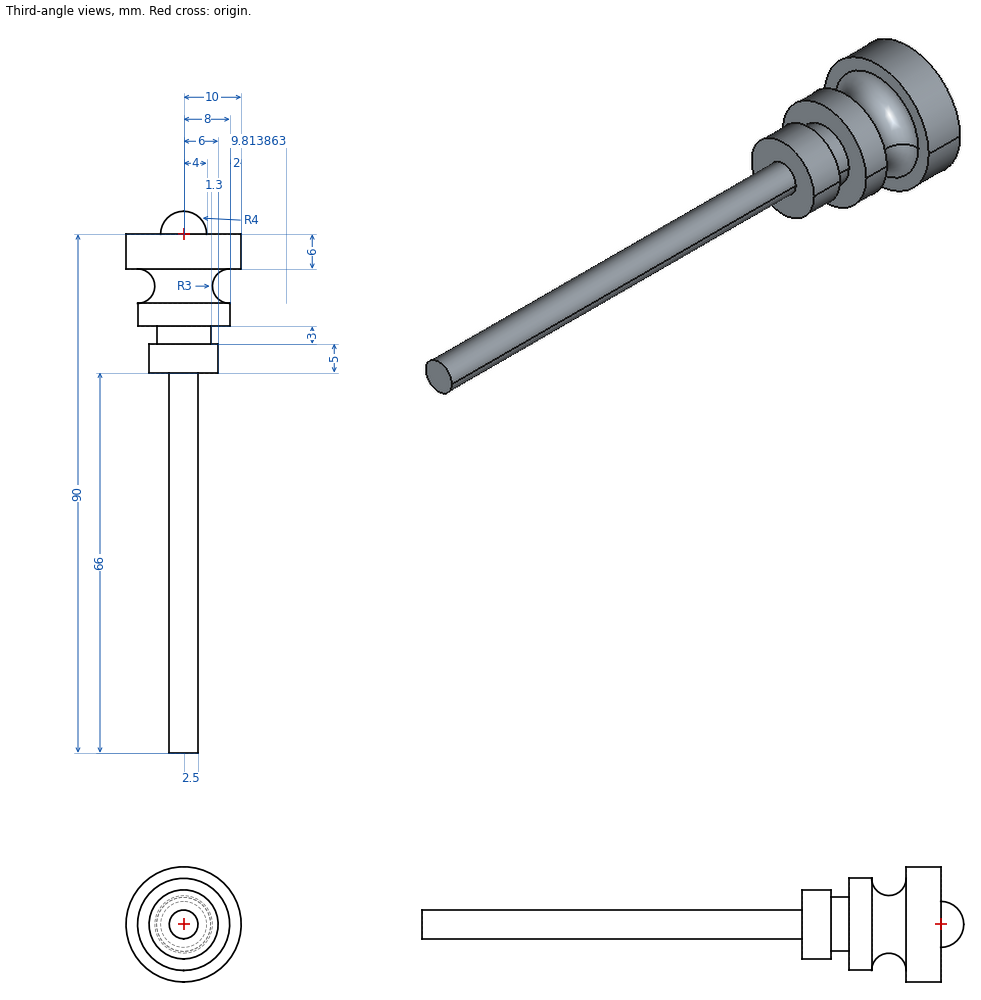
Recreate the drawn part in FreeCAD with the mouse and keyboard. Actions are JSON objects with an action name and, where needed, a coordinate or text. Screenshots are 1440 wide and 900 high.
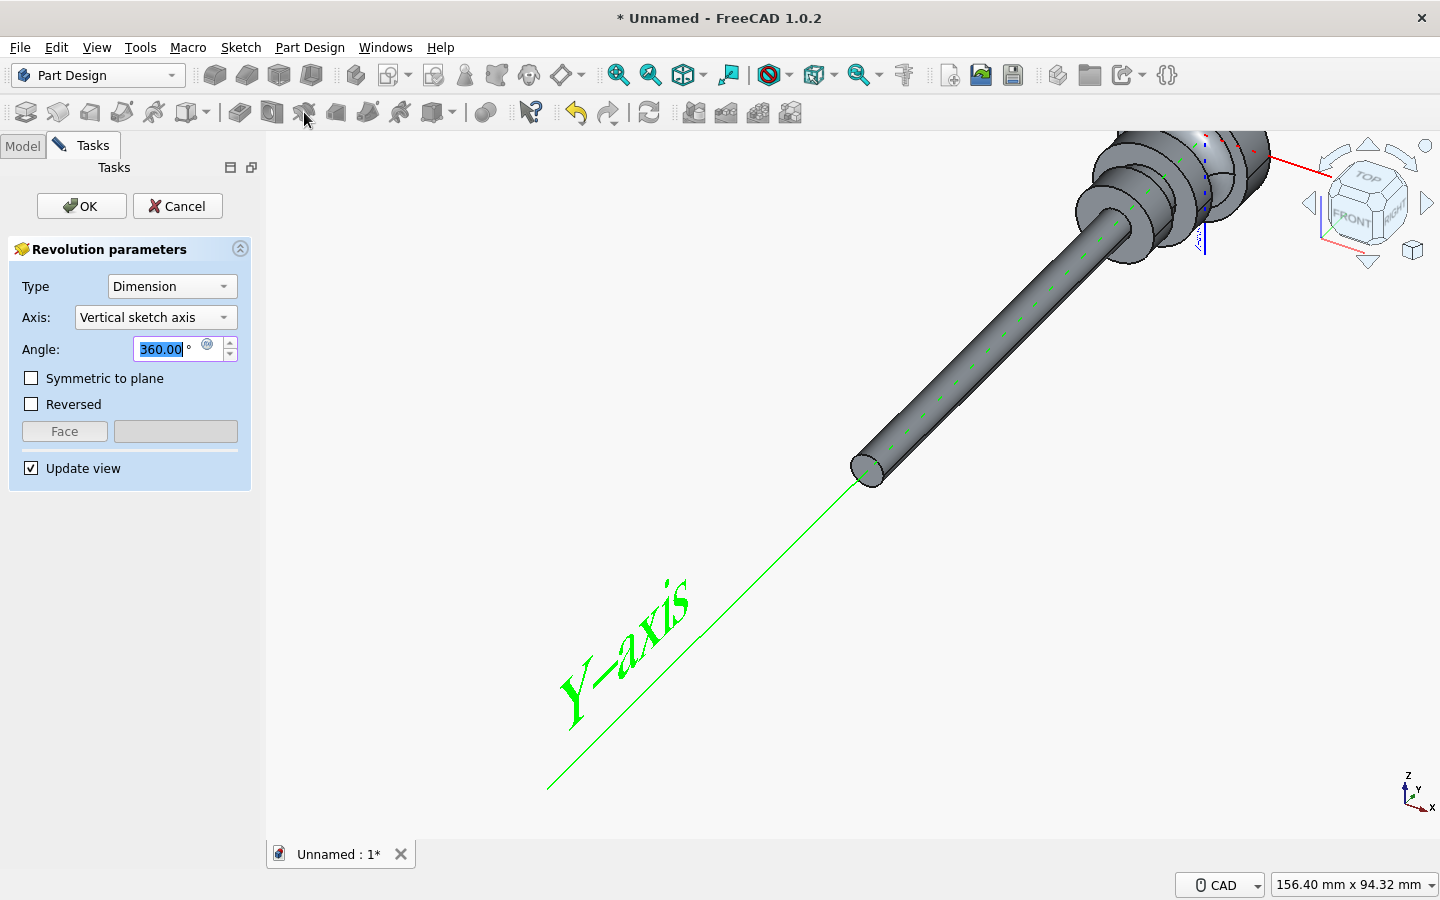
{"action": "left_click", "coordinate": [82, 206]}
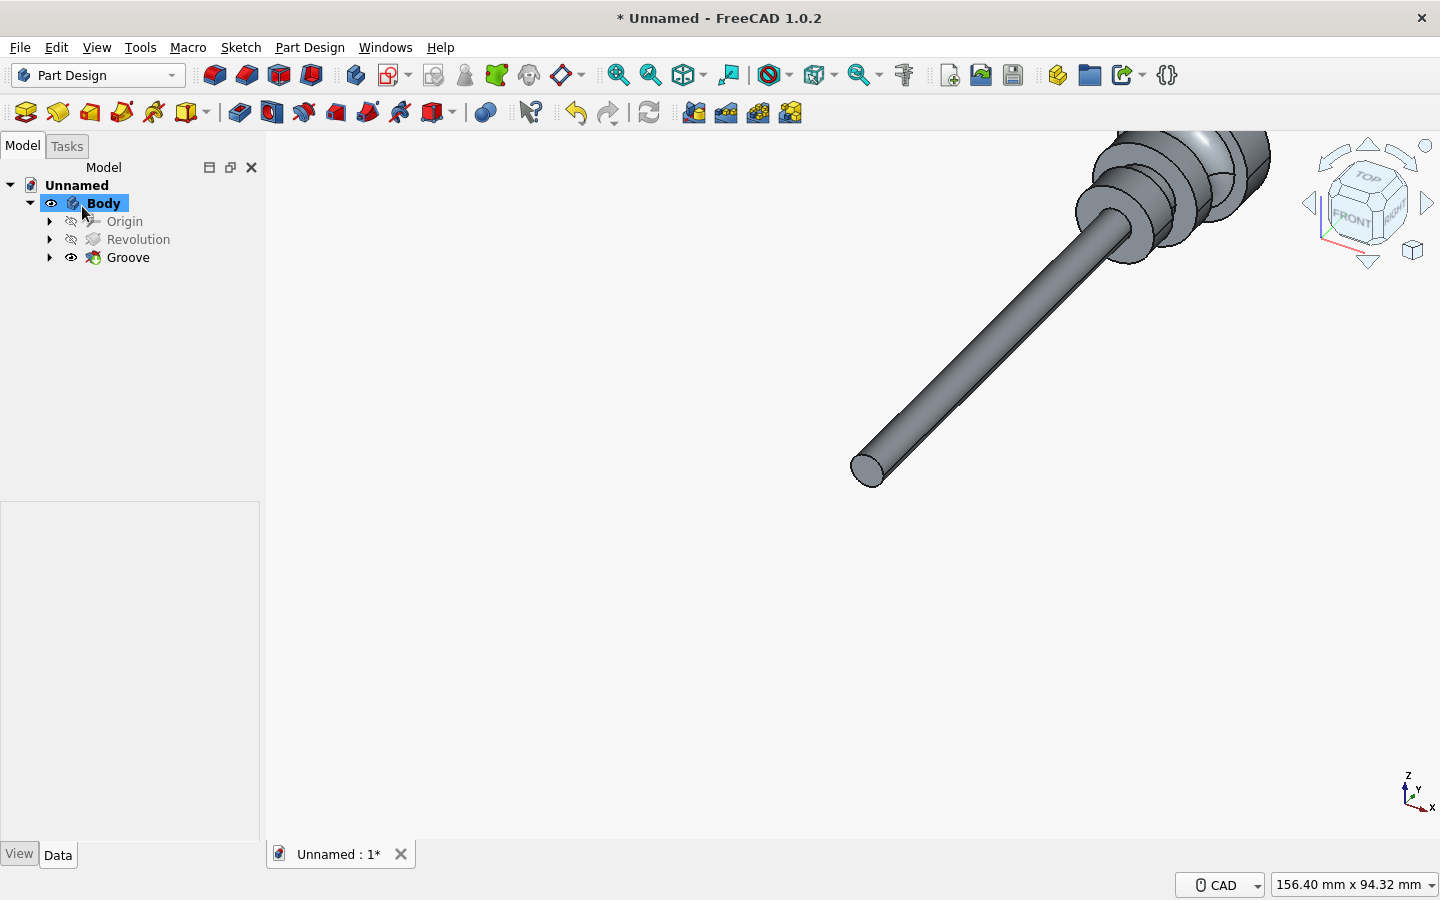
{"action": "left_click", "coordinate": [620, 76]}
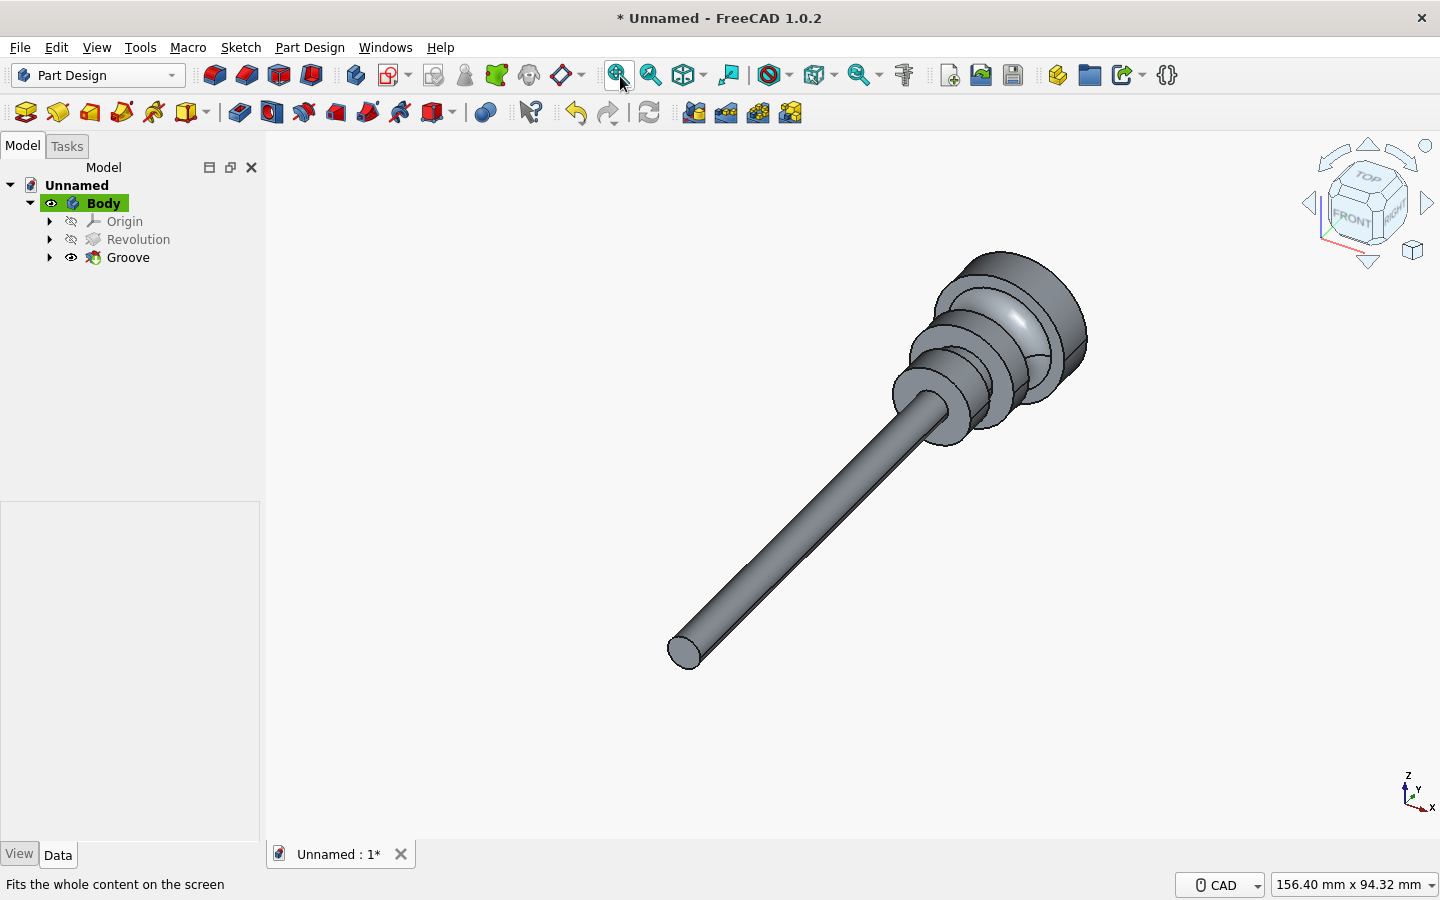
{"action": "left_click", "coordinate": [388, 76]}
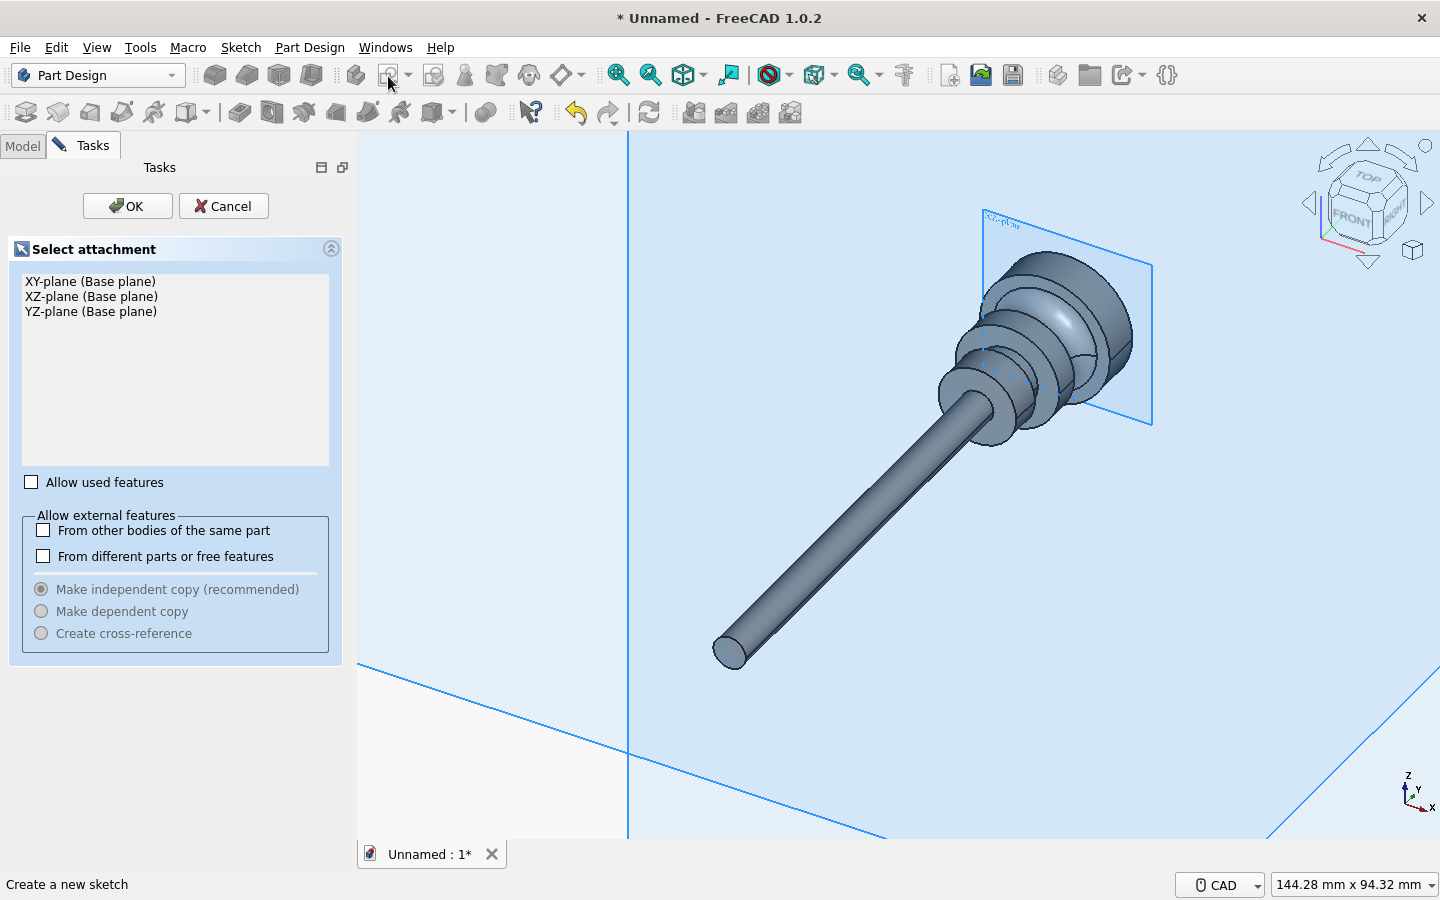
{"action": "left_click", "coordinate": [82, 282]}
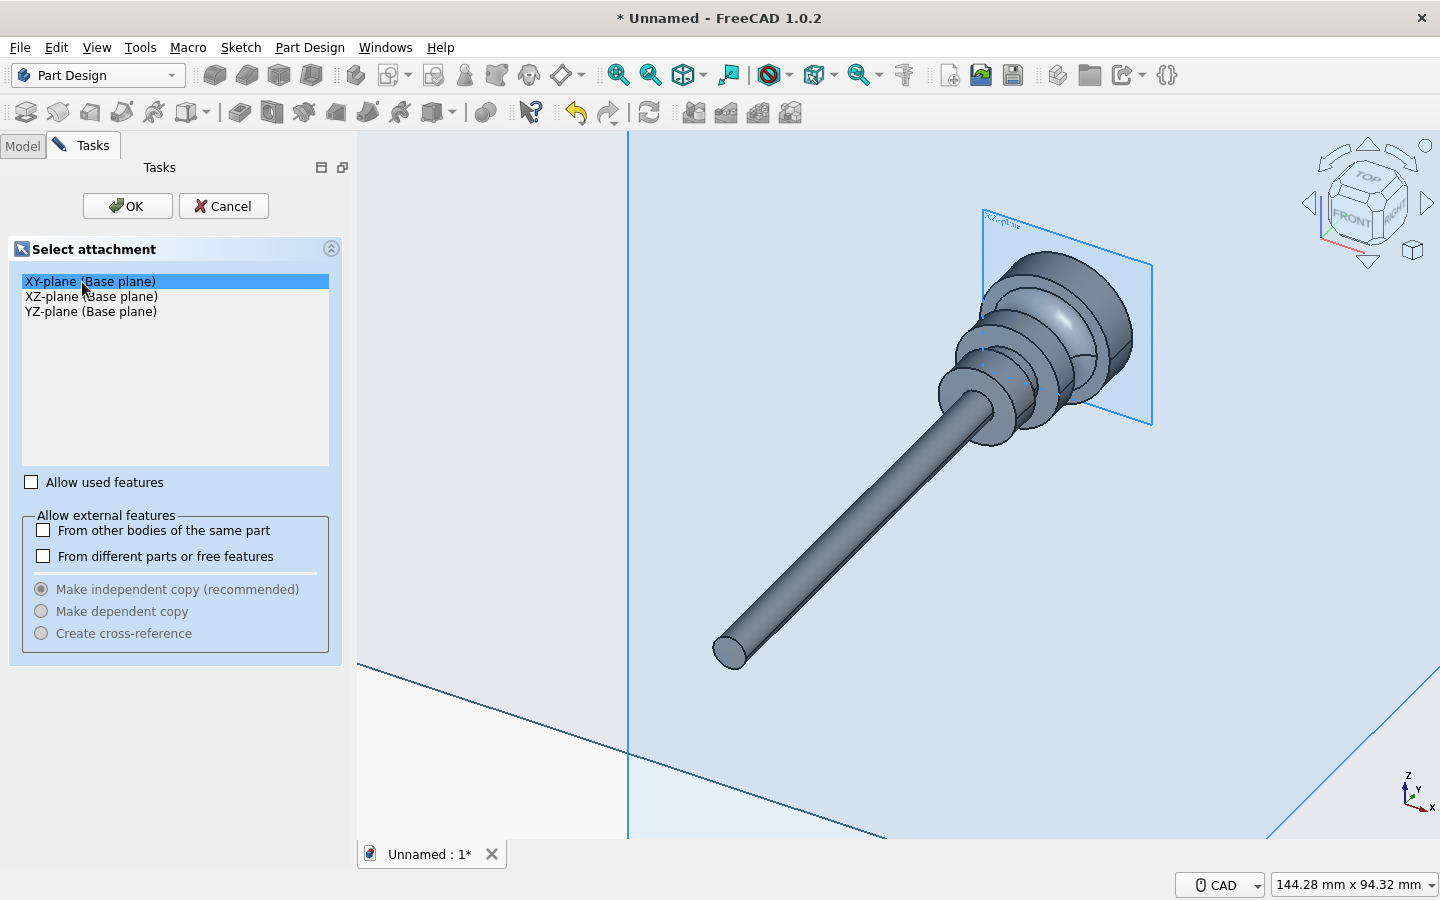
{"action": "left_click", "coordinate": [128, 206]}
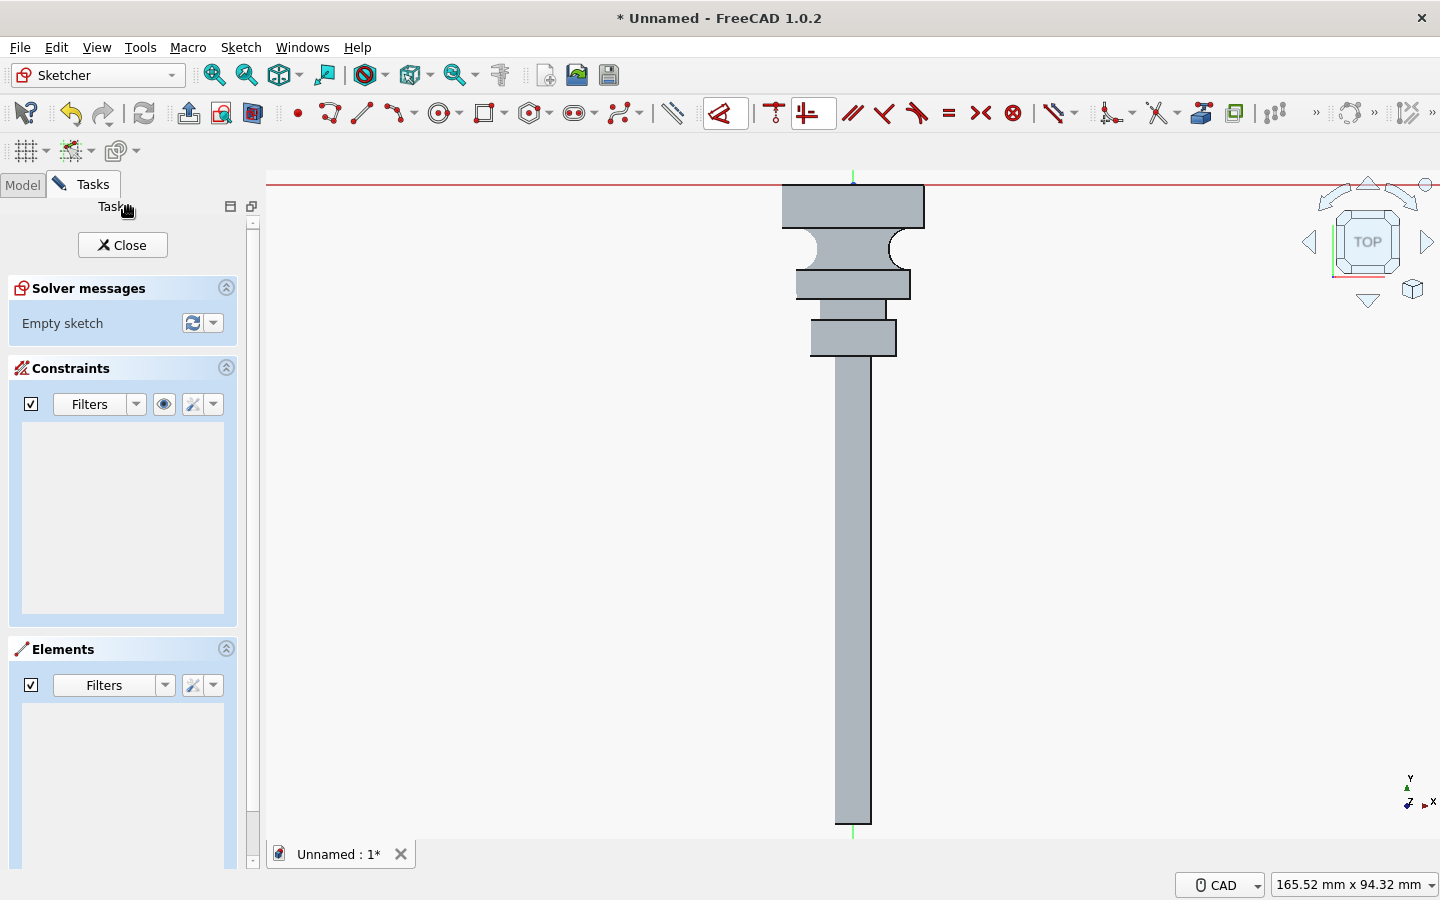
{"action": "left_click", "coordinate": [254, 114]}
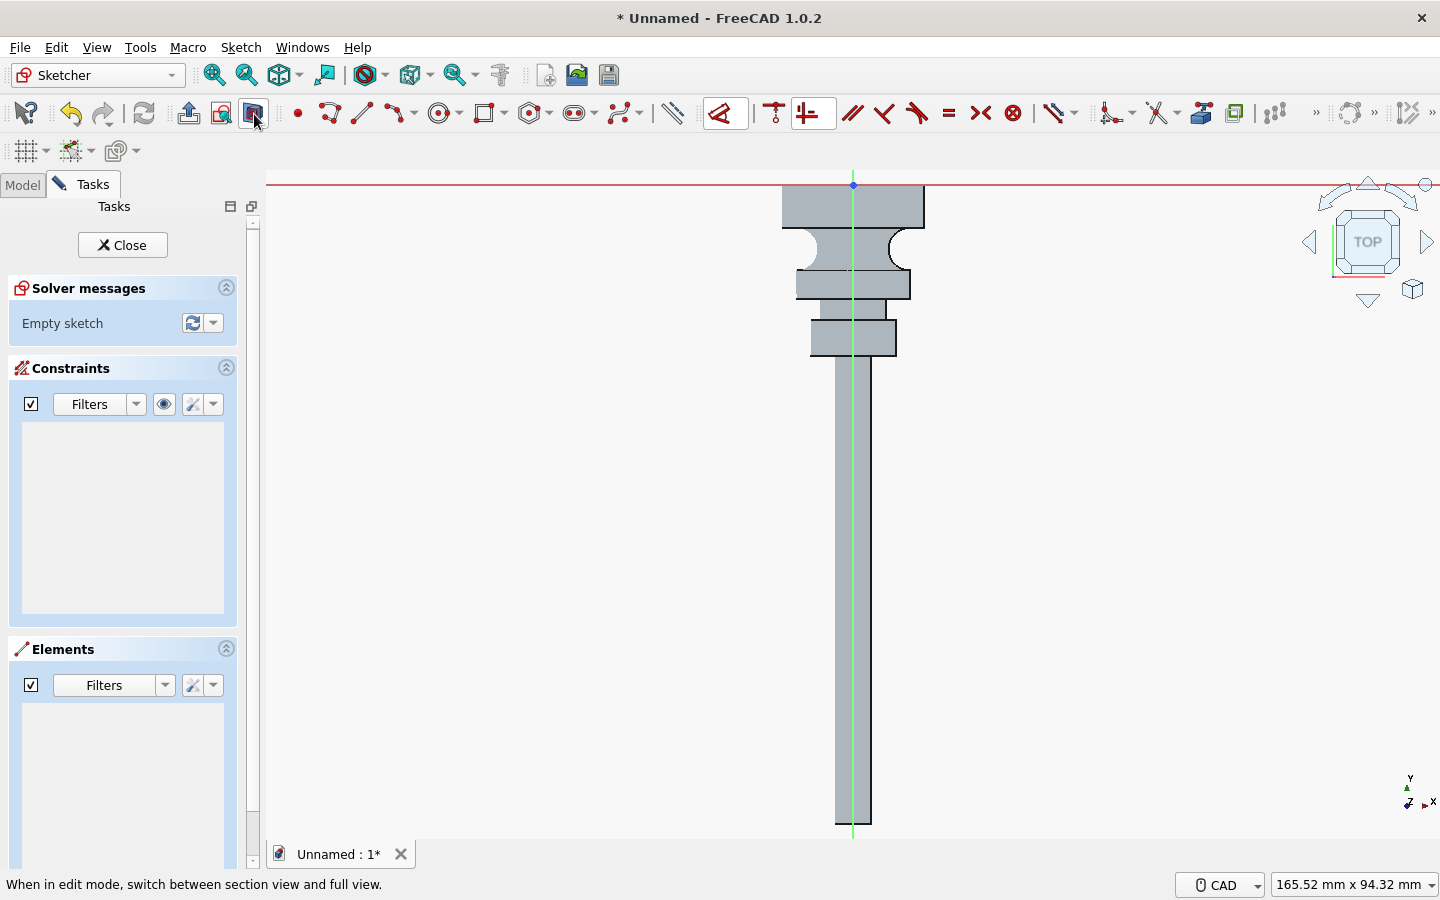
{"action": "scroll", "coordinate": [784, 504], "scroll_direction": "down", "scroll_amount": 5}